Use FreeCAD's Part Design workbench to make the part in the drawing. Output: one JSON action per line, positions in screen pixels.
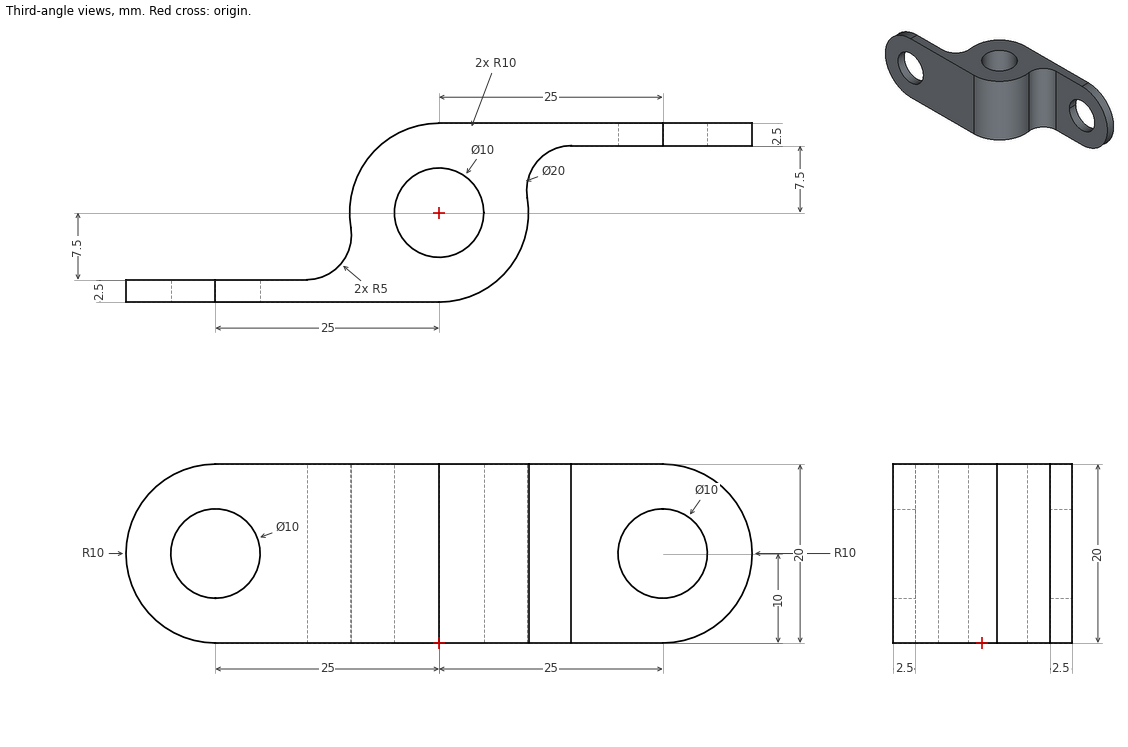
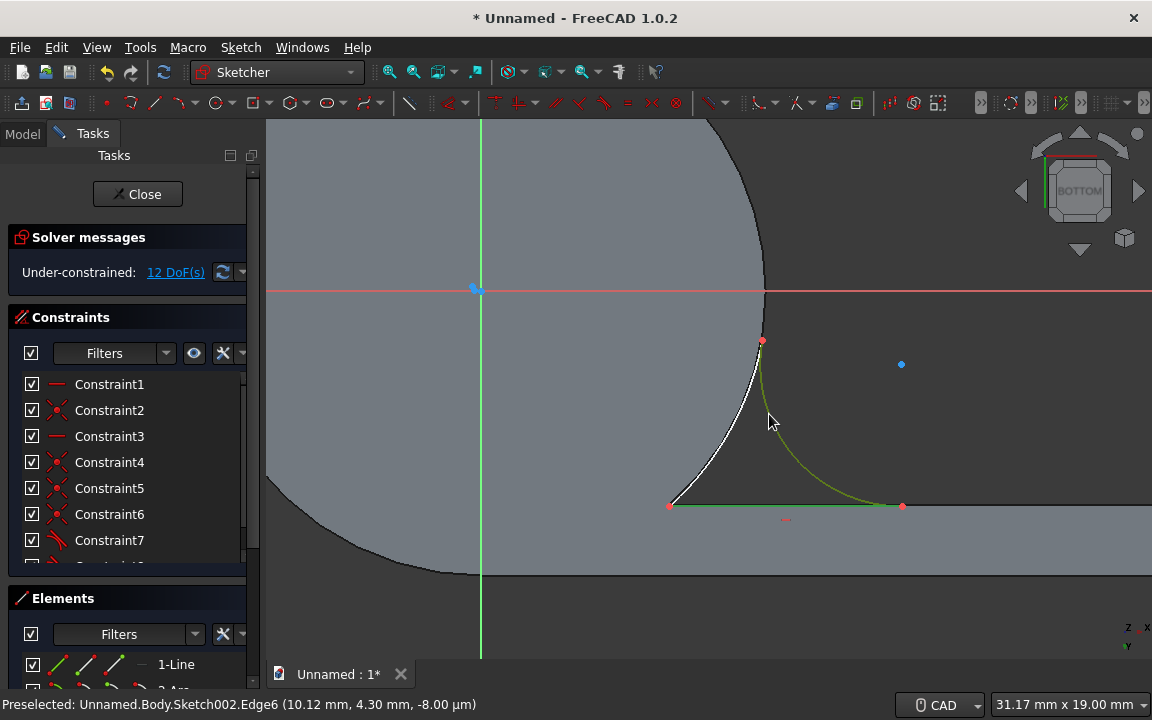
{"action": "key", "text": "t"}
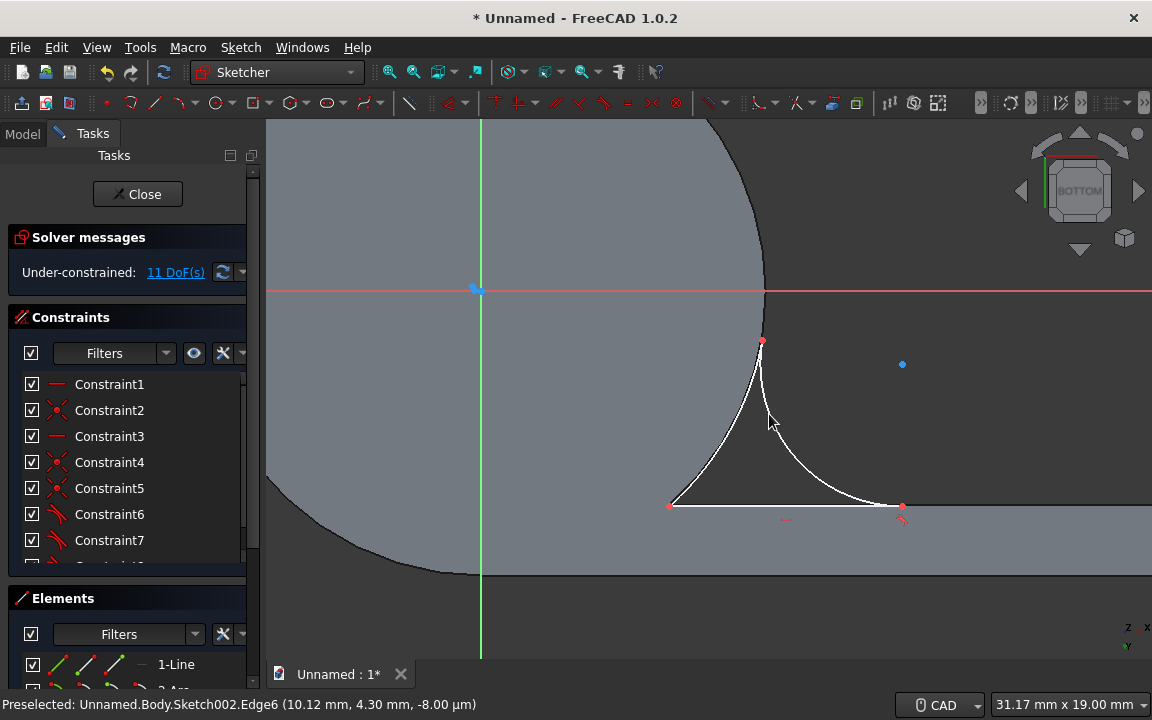
{"action": "left_click", "coordinate": [709, 464]}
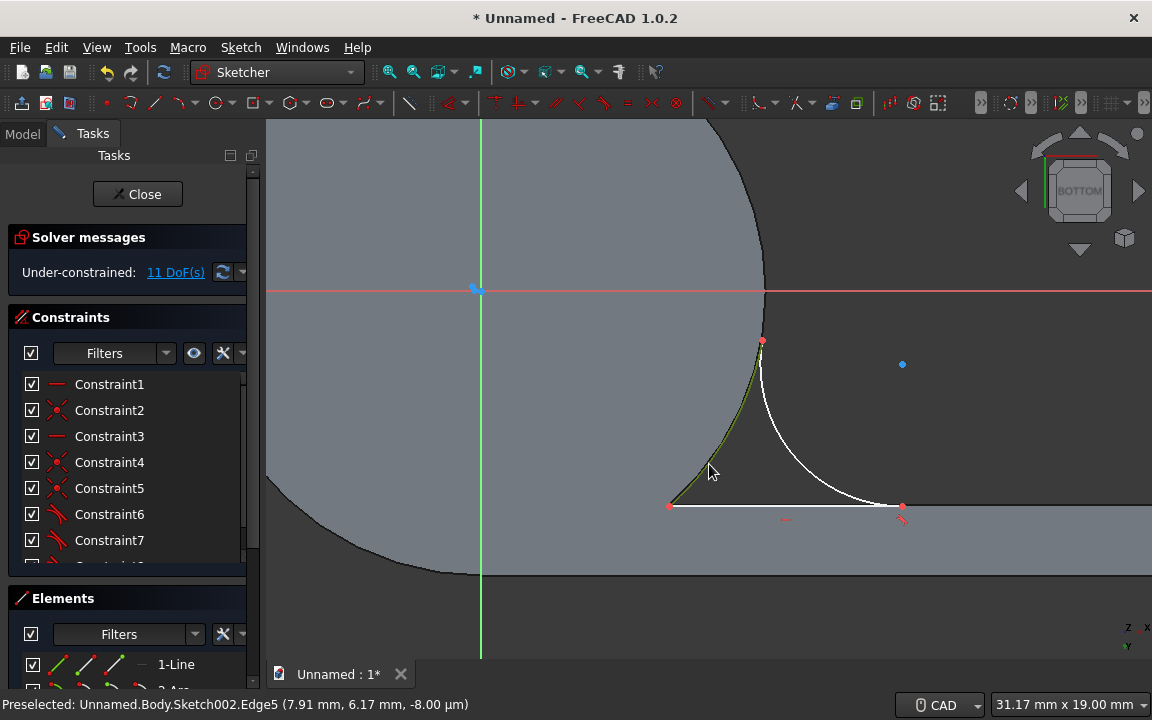
{"action": "left_click", "coordinate": [769, 414]}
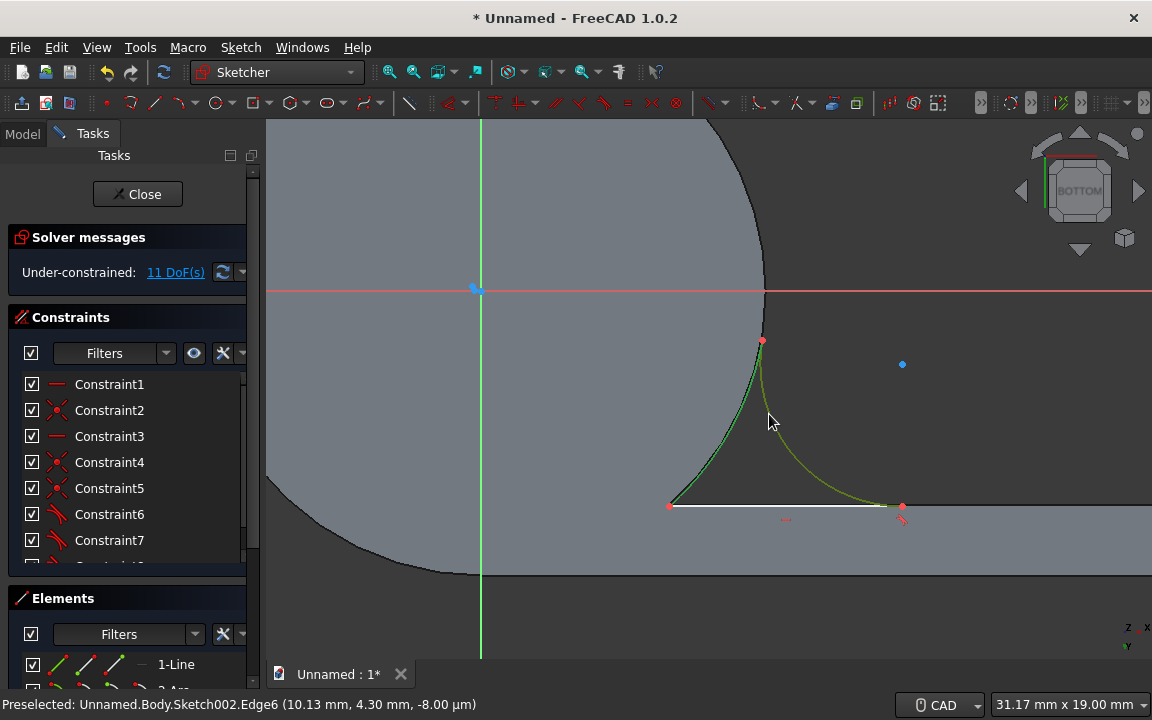
{"action": "left_click", "coordinate": [604, 104]}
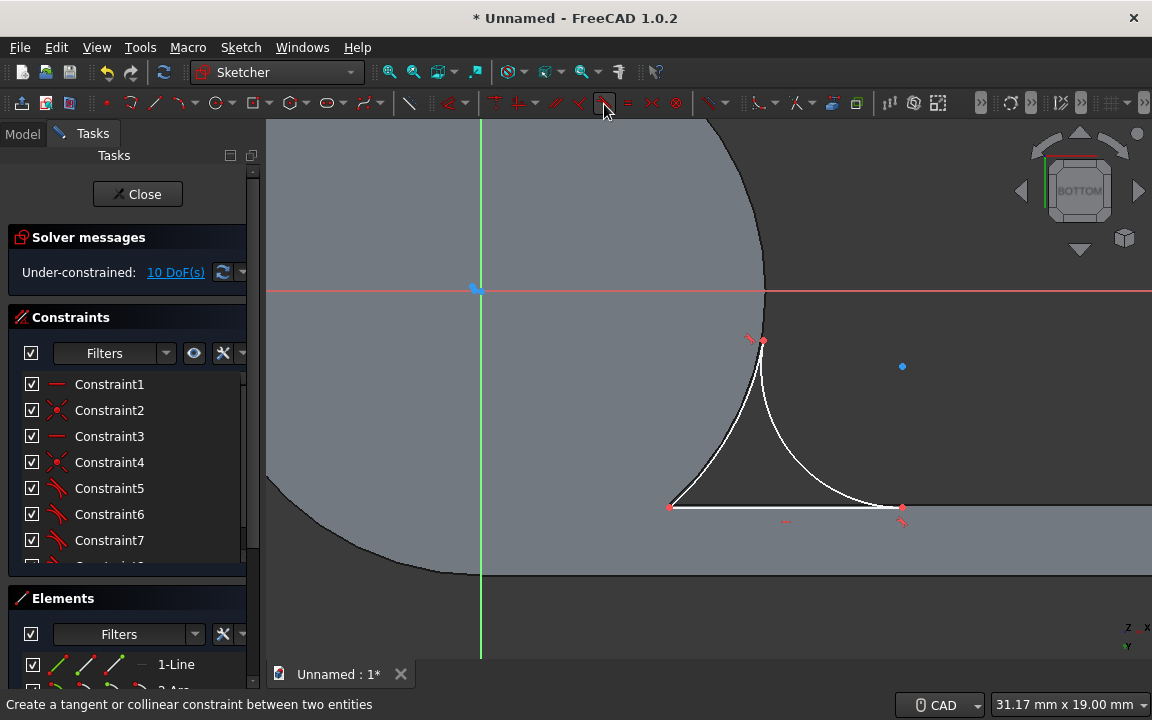
{"action": "scroll", "coordinate": [834, 508], "scroll_direction": "down", "scroll_amount": 3}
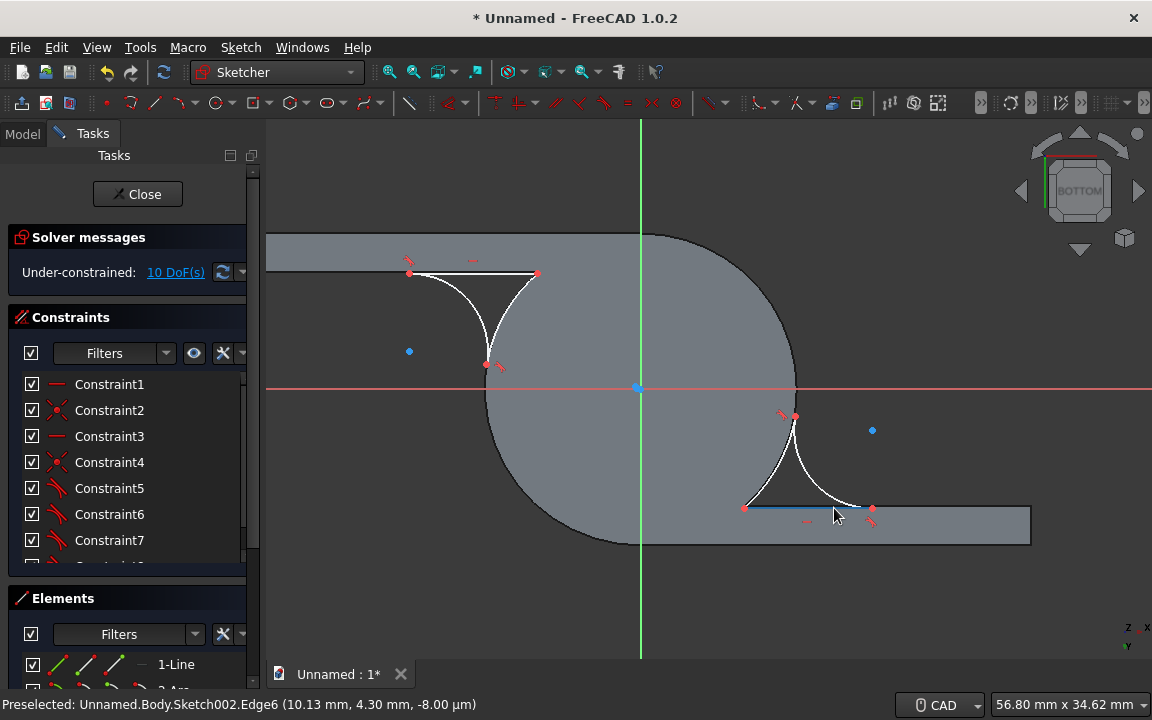
{"action": "left_click", "coordinate": [516, 297]}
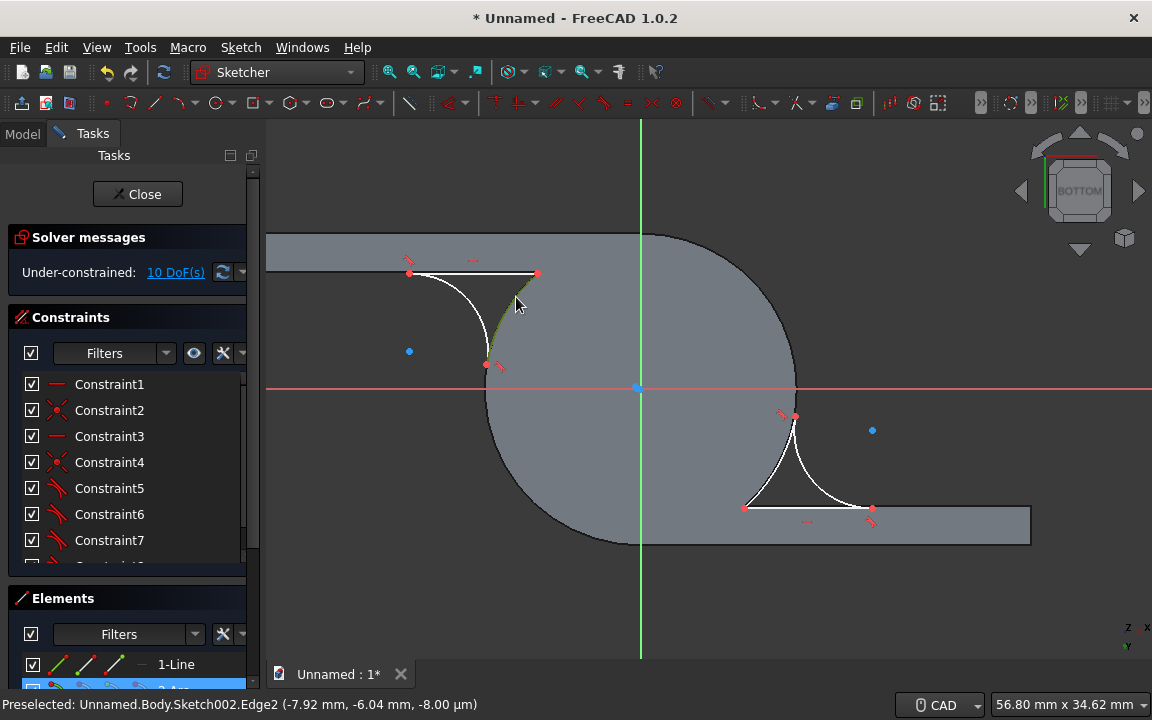
{"action": "left_click", "coordinate": [766, 485]}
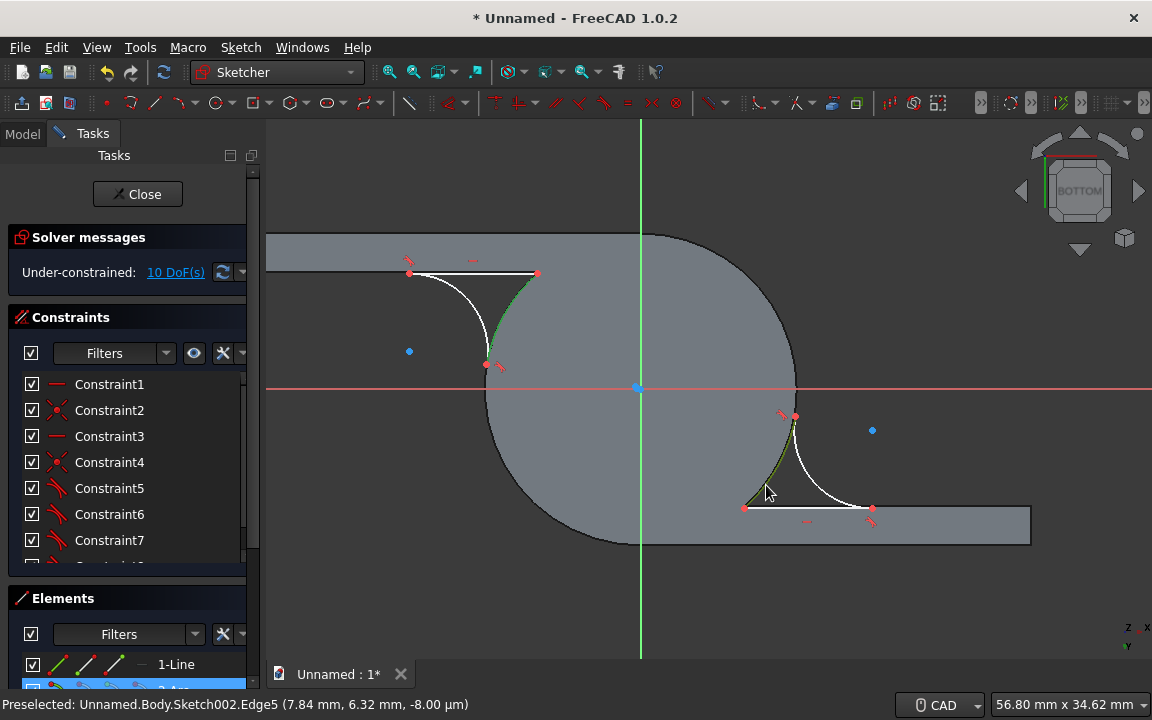
{"action": "left_click", "coordinate": [496, 104]}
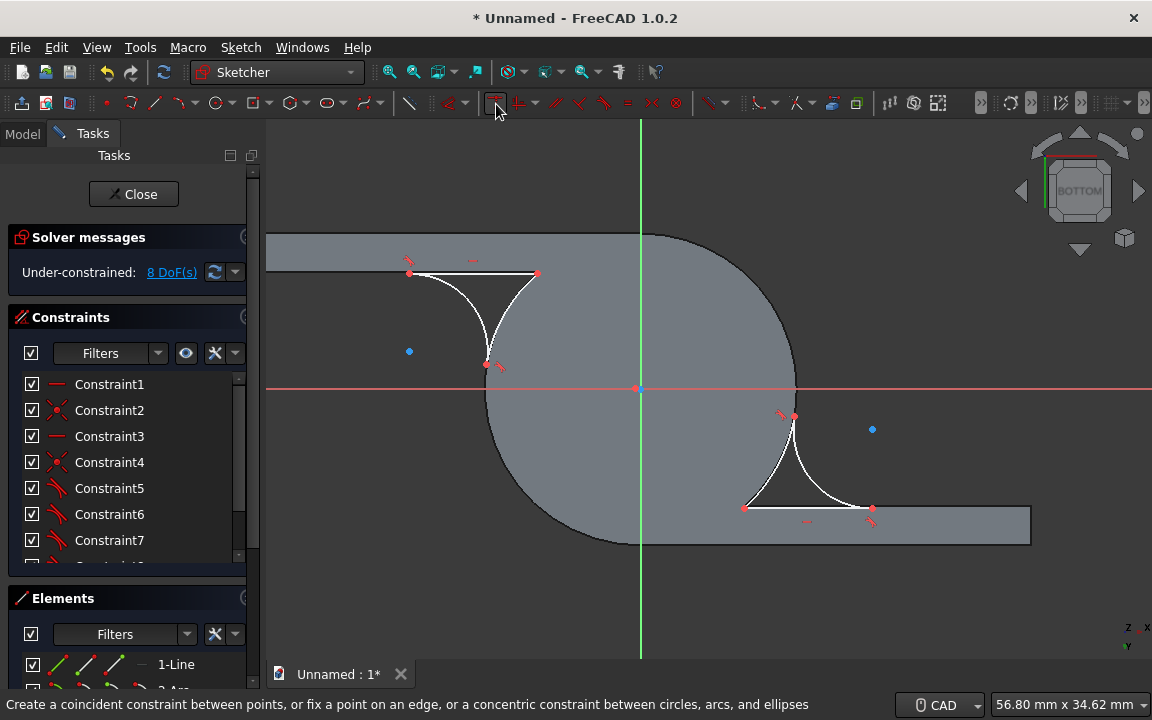
{"action": "left_click_drag", "start_coordinate": [626, 379], "coordinate": [651, 399]}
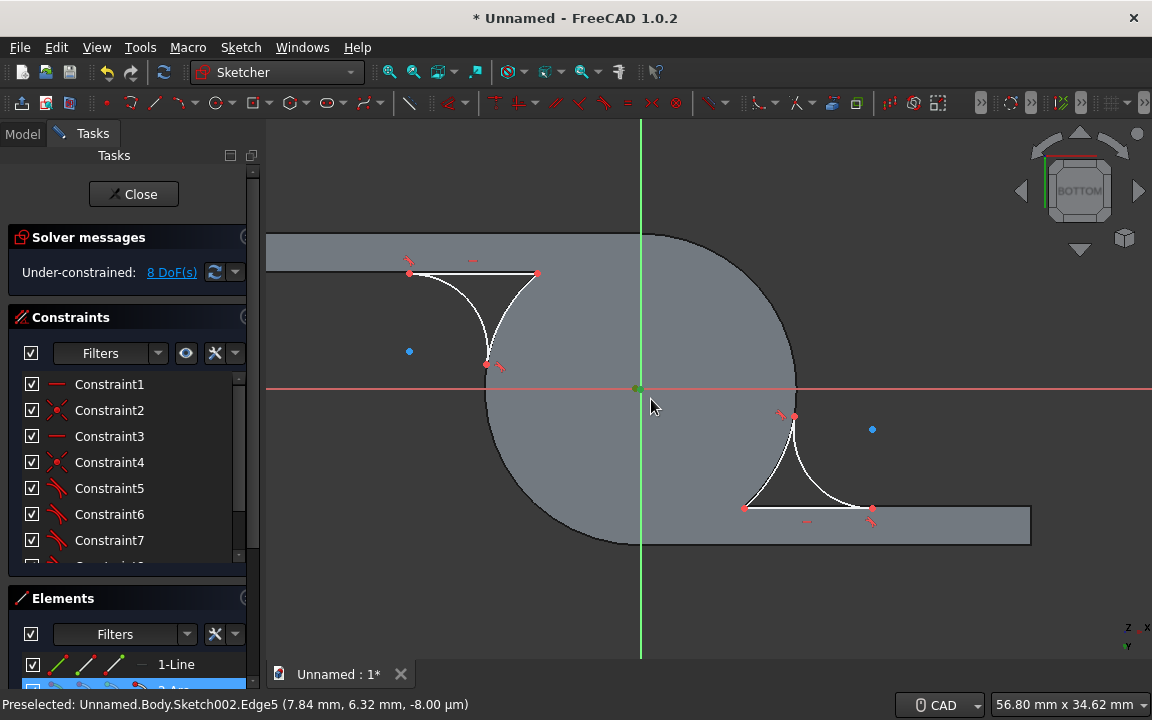
{"action": "key", "text": "c"}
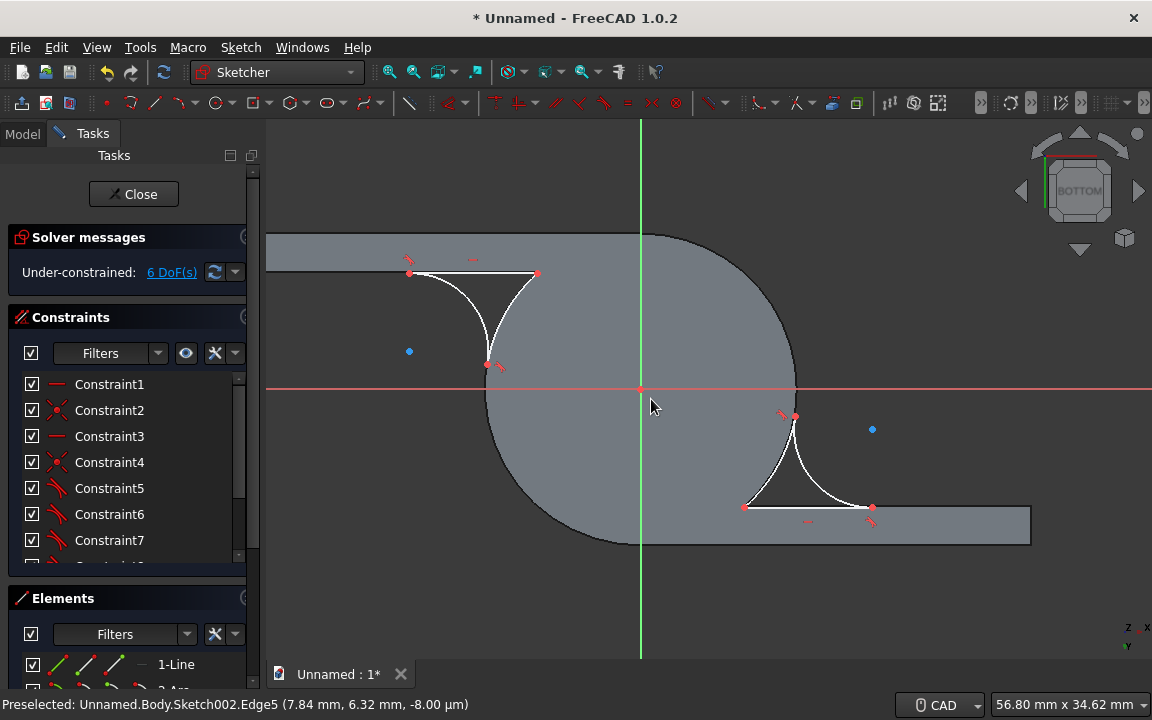
{"action": "left_click", "coordinate": [516, 297]}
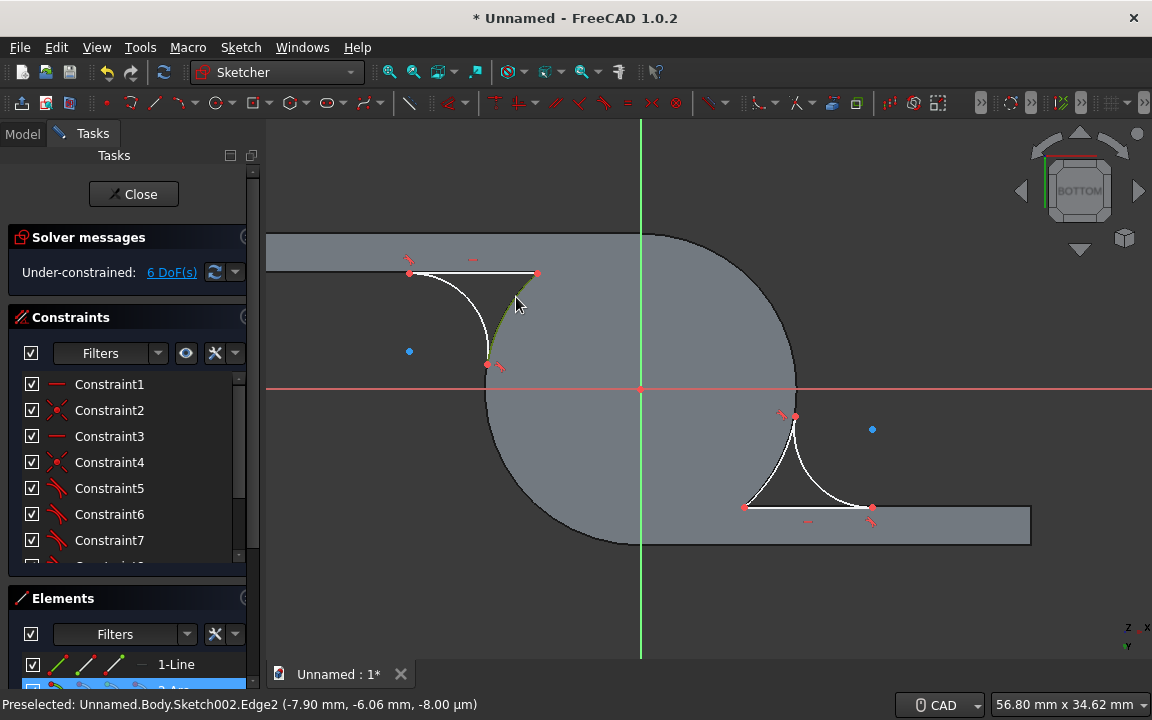
{"action": "left_click", "coordinate": [766, 484]}